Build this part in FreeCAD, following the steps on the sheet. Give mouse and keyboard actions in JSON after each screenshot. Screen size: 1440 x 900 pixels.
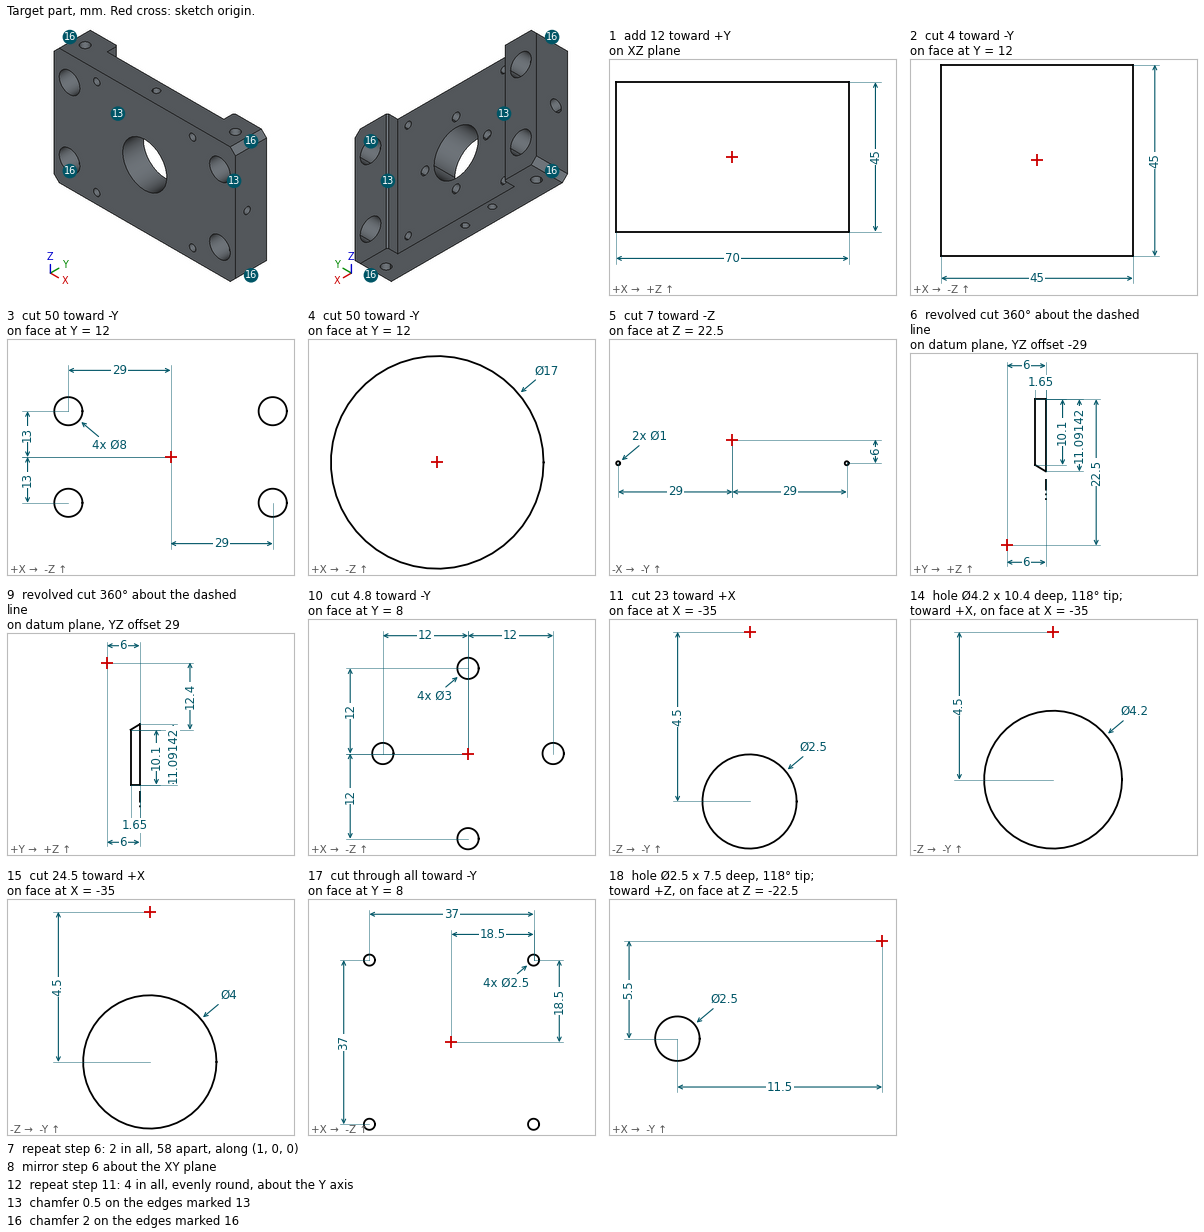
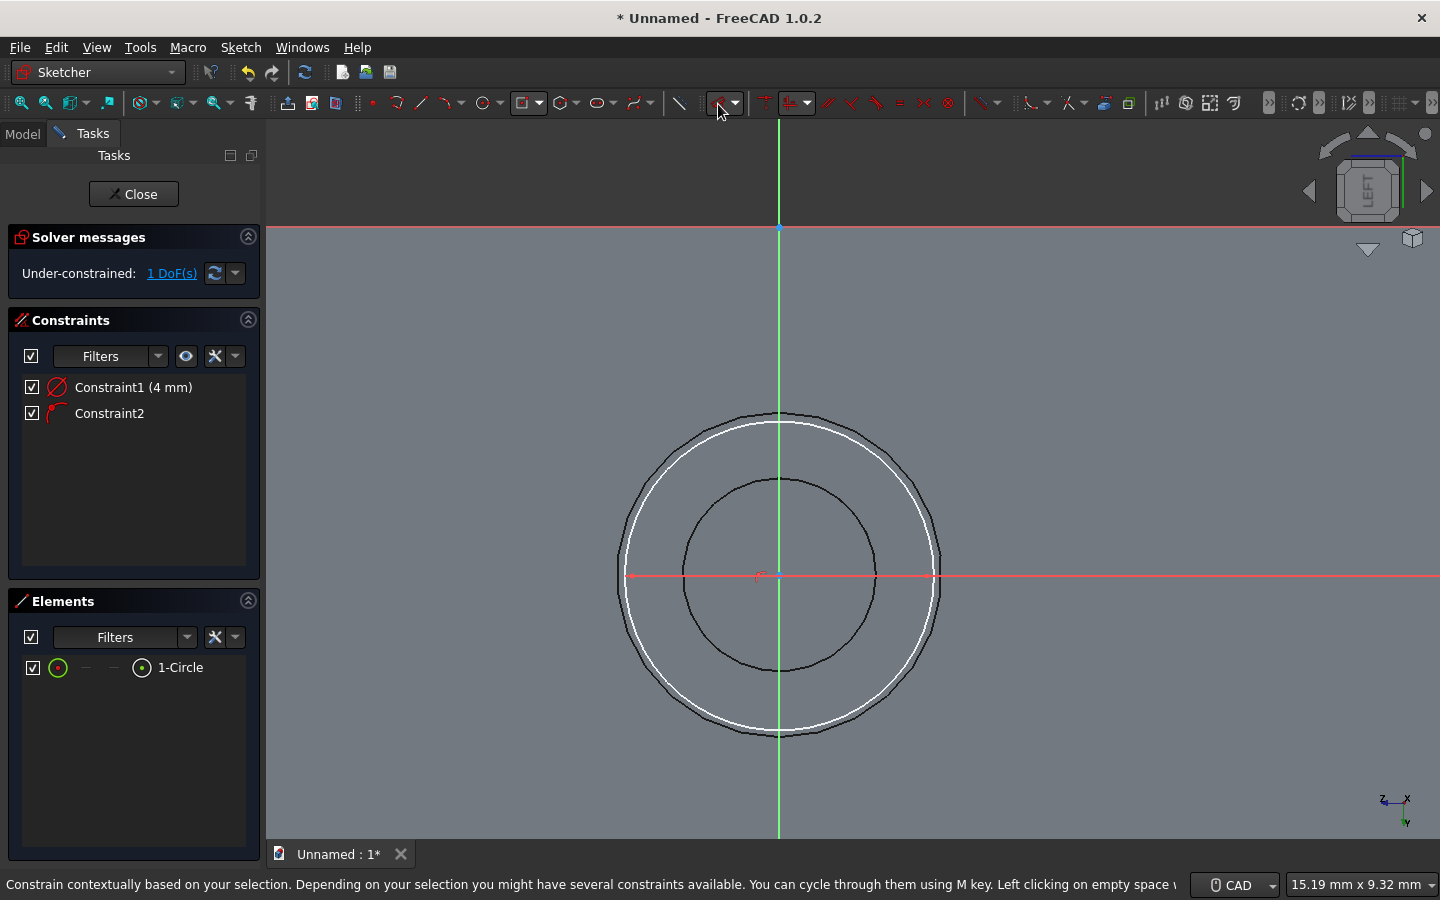
{"action": "left_click", "coordinate": [779, 576]}
{"action": "left_click", "coordinate": [813, 402]}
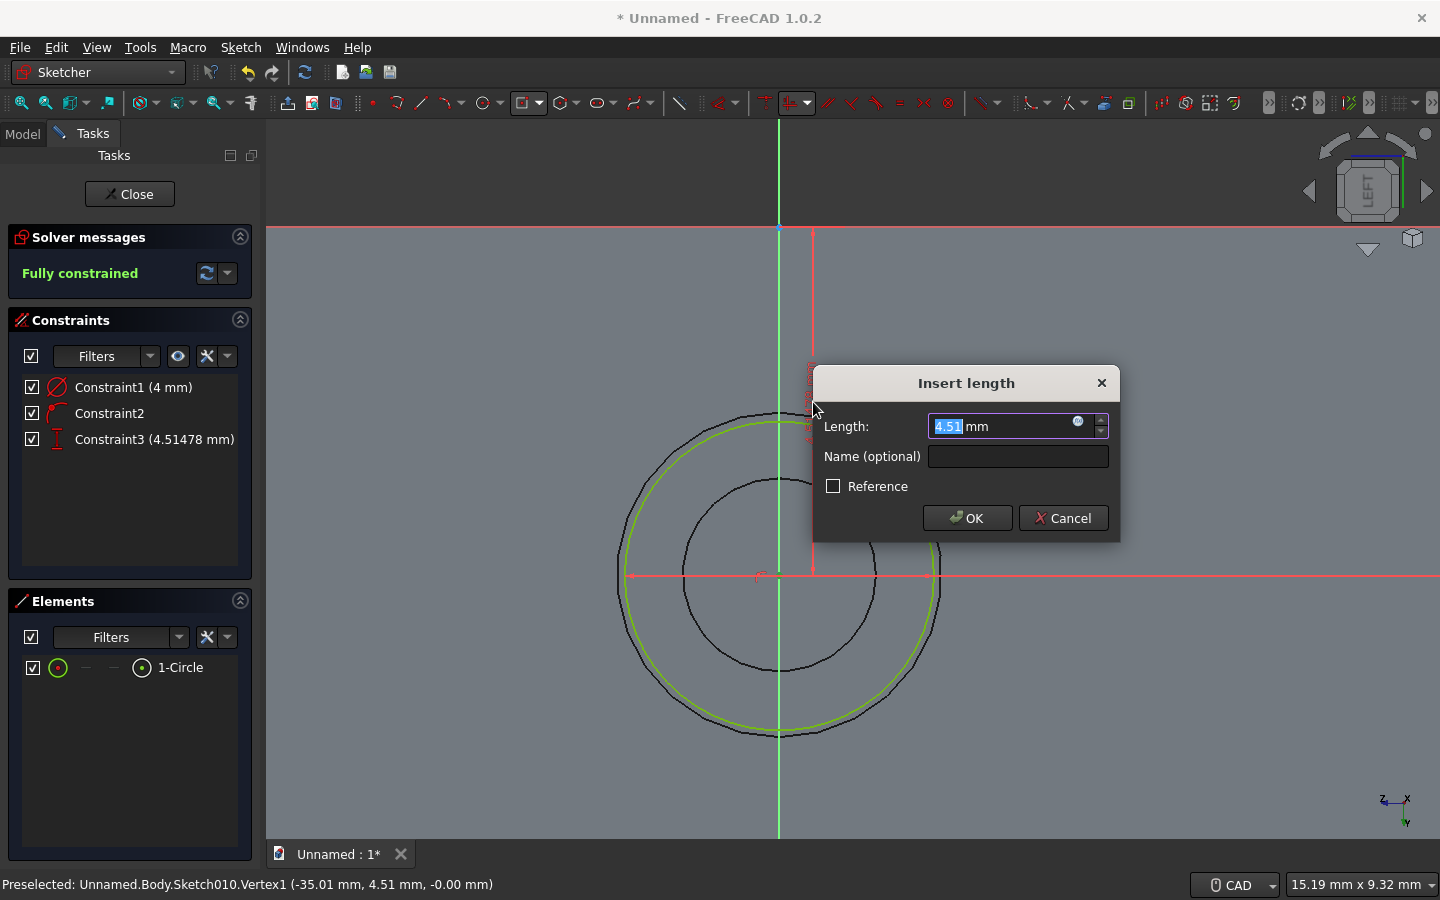
{"action": "type", "text": "4.5"}
{"action": "key", "text": "Return"}
{"action": "key", "text": "Escape"}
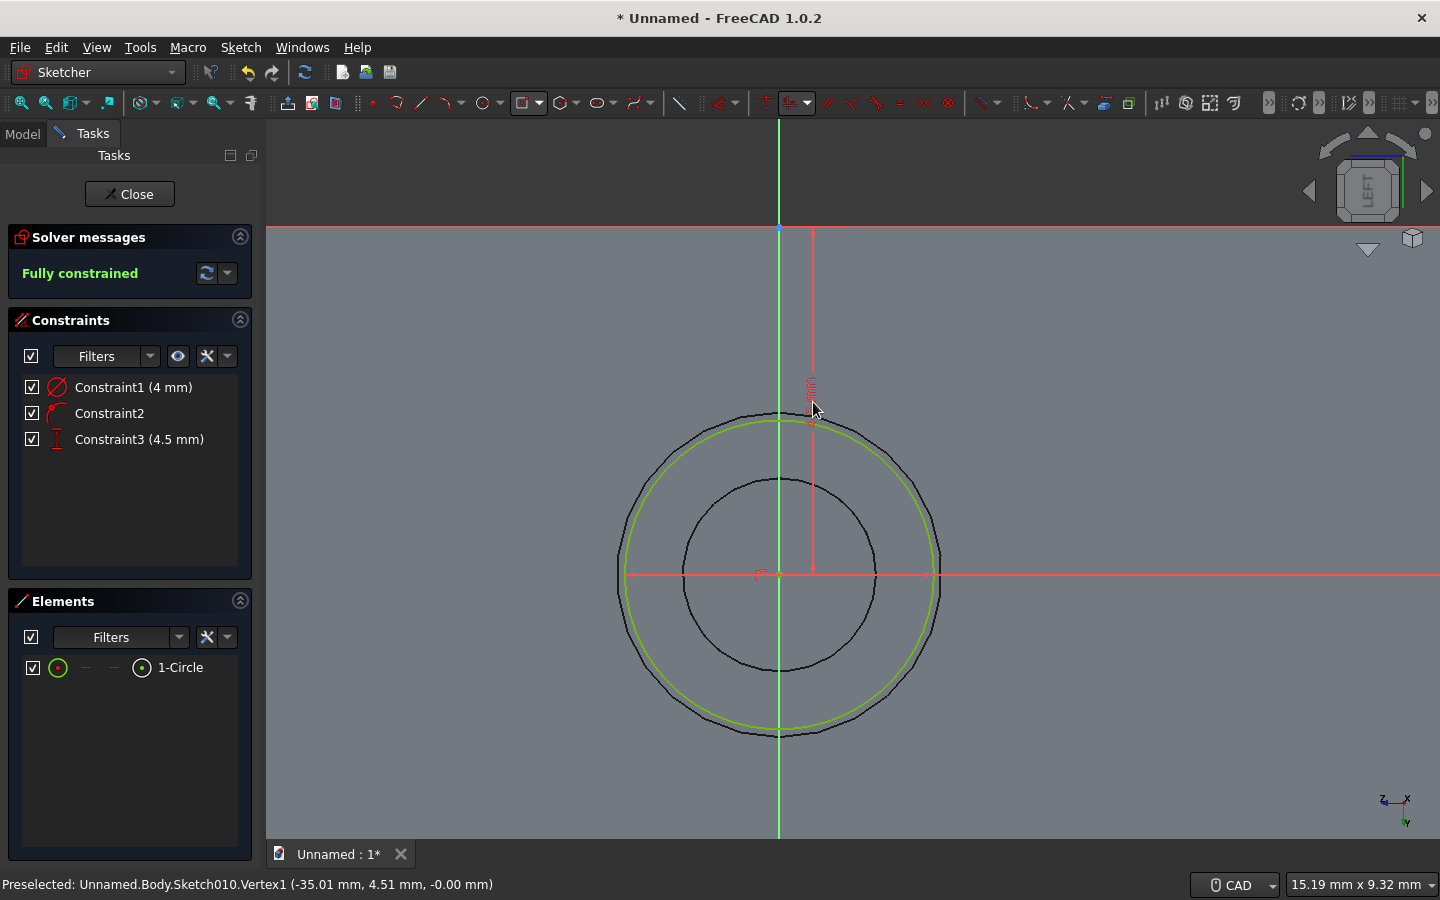
{"action": "left_click", "coordinate": [130, 194]}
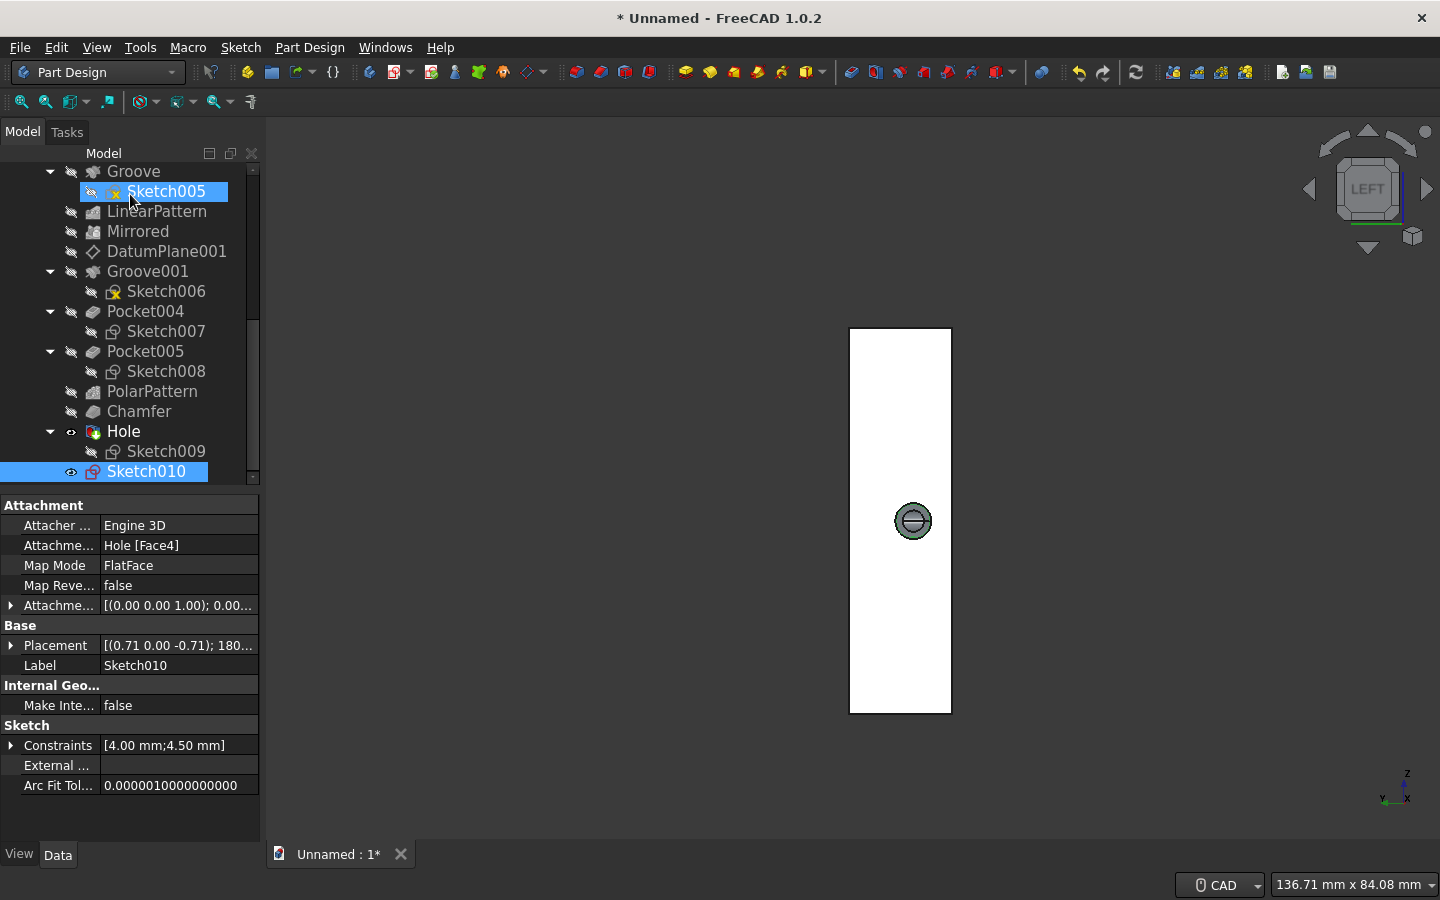
{"action": "left_click", "coordinate": [852, 72]}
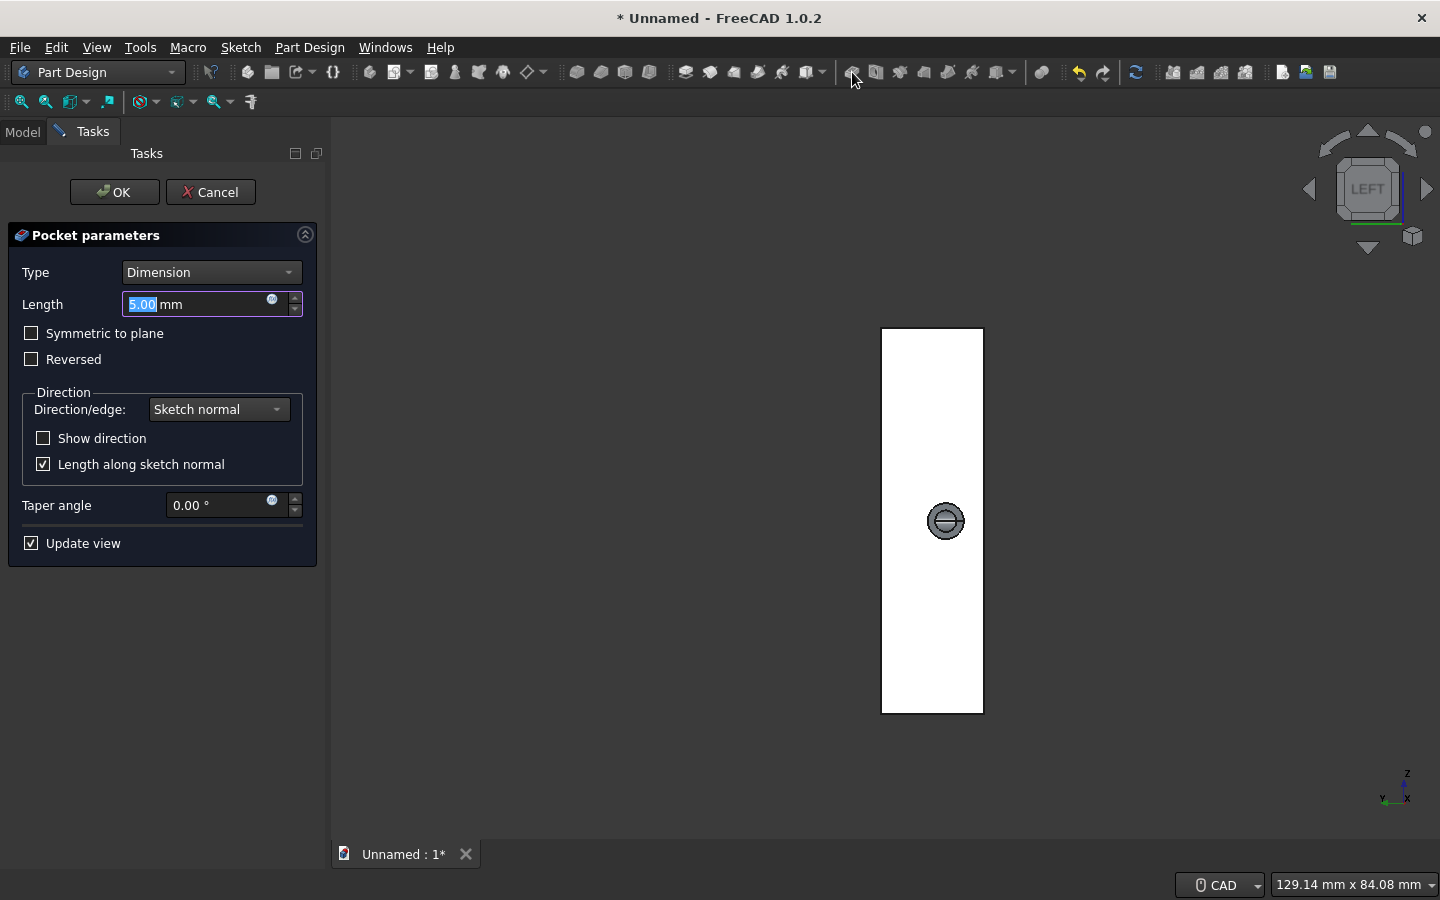
{"action": "type", "text": "24.5"}
{"action": "key", "text": "Tab"}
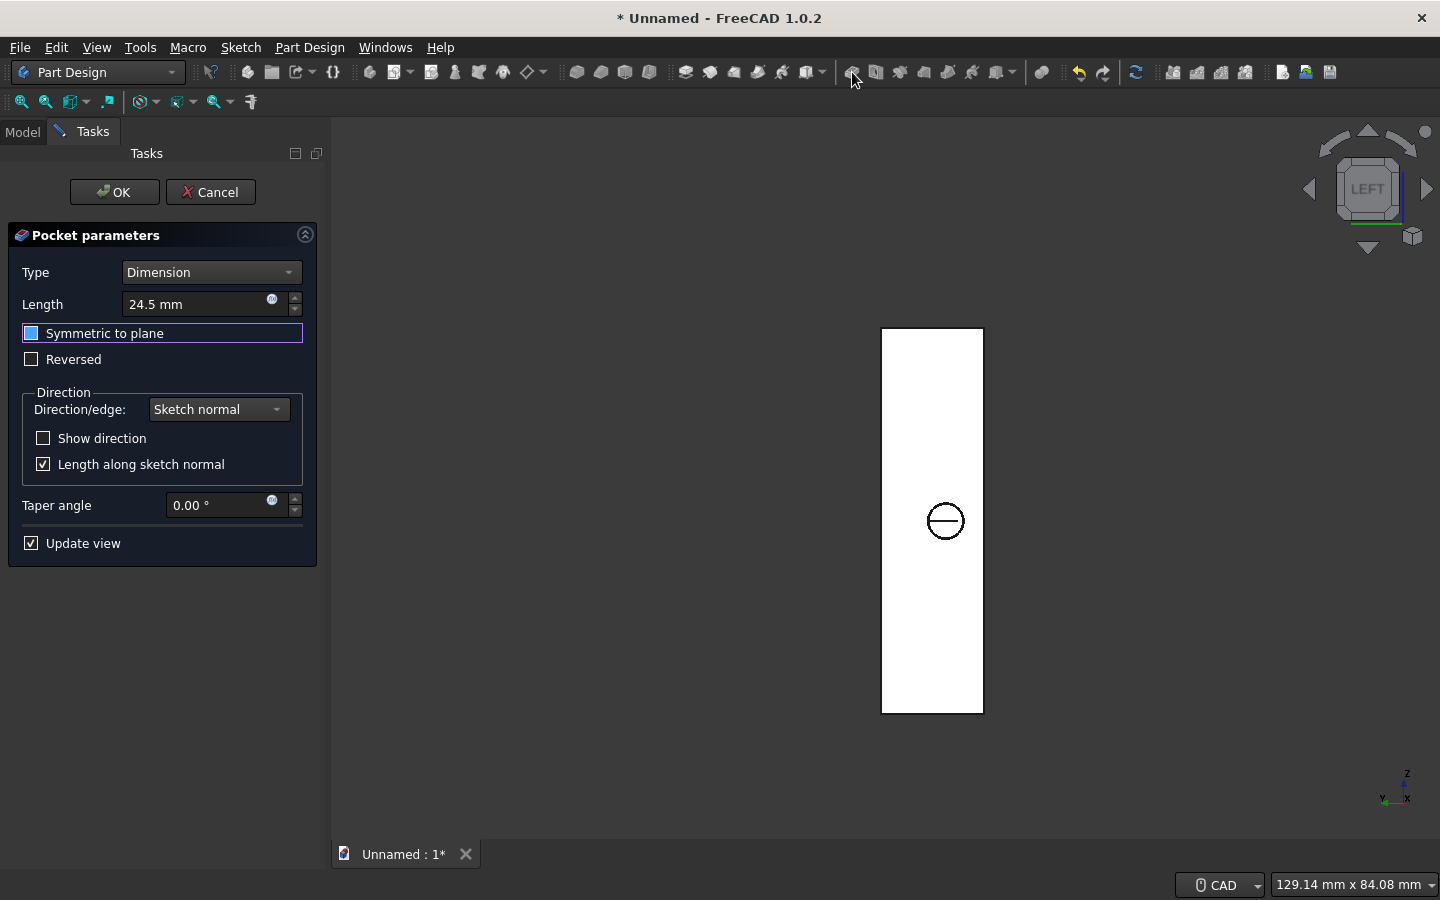
{"action": "left_click", "coordinate": [115, 192]}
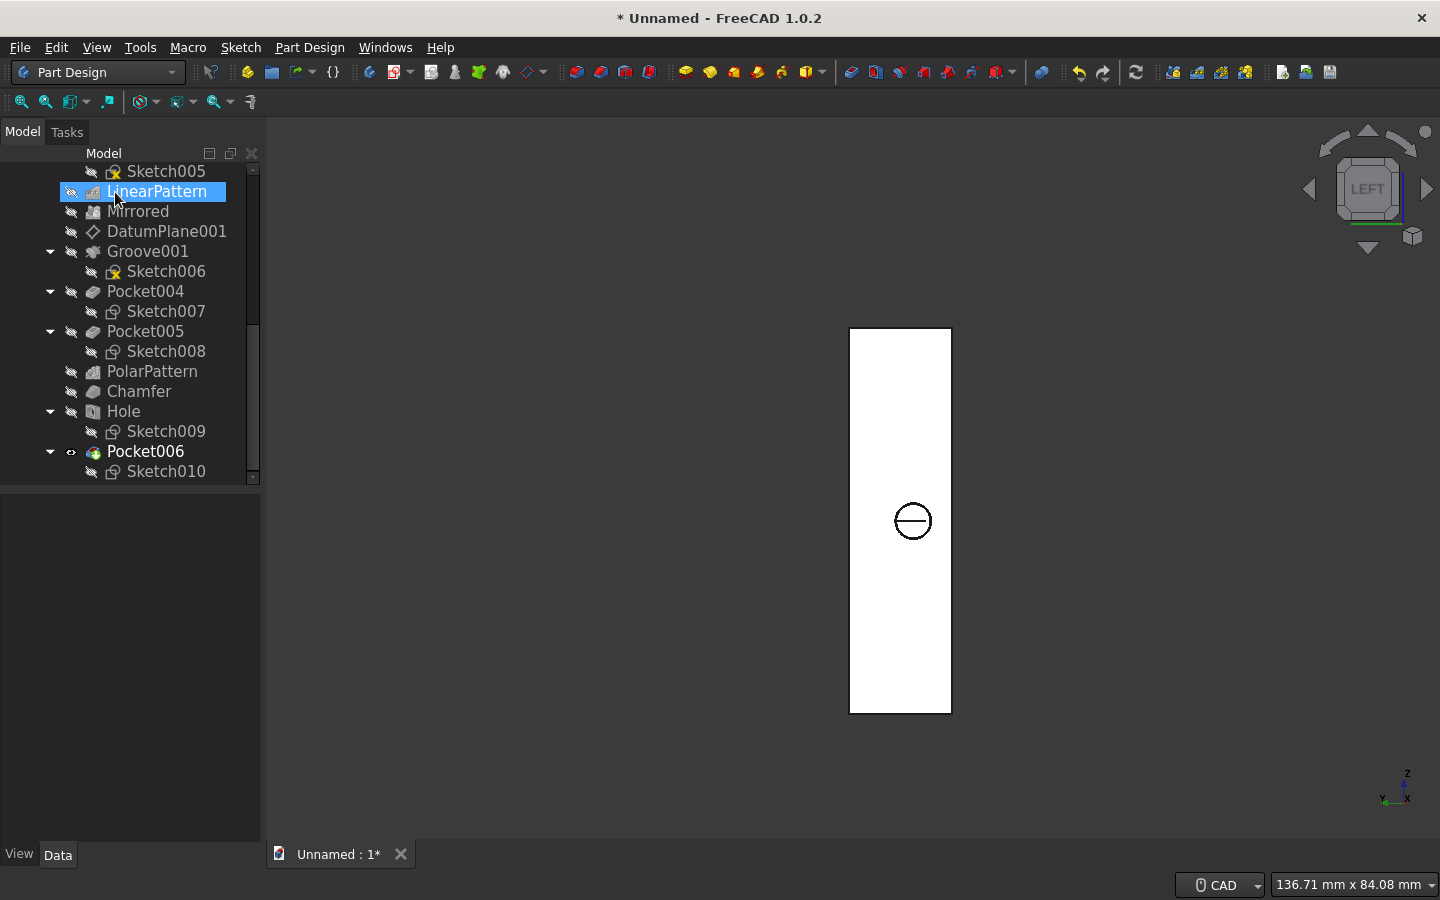
{"action": "left_click", "coordinate": [900, 327]}